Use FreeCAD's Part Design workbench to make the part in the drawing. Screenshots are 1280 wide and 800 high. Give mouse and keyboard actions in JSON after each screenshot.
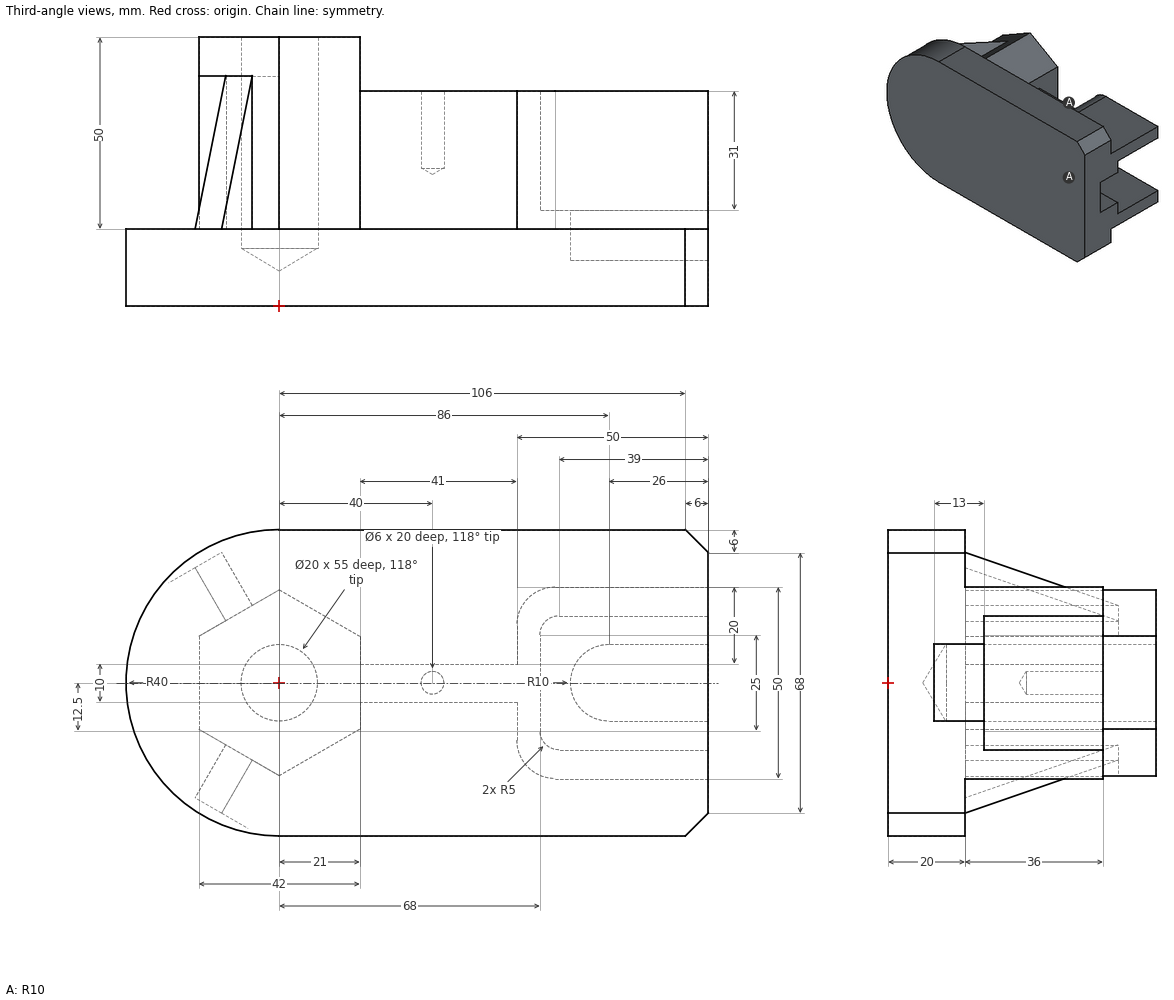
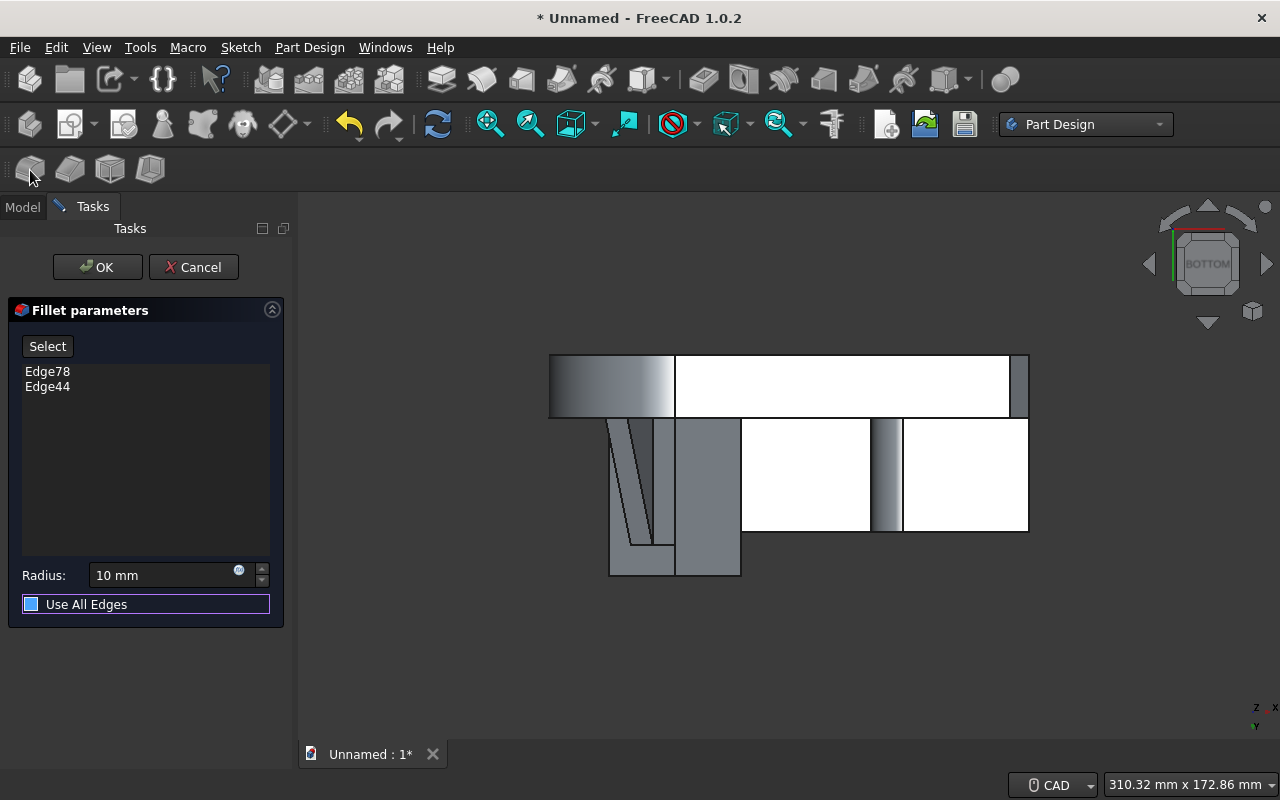
{"action": "left_click", "coordinate": [98, 267]}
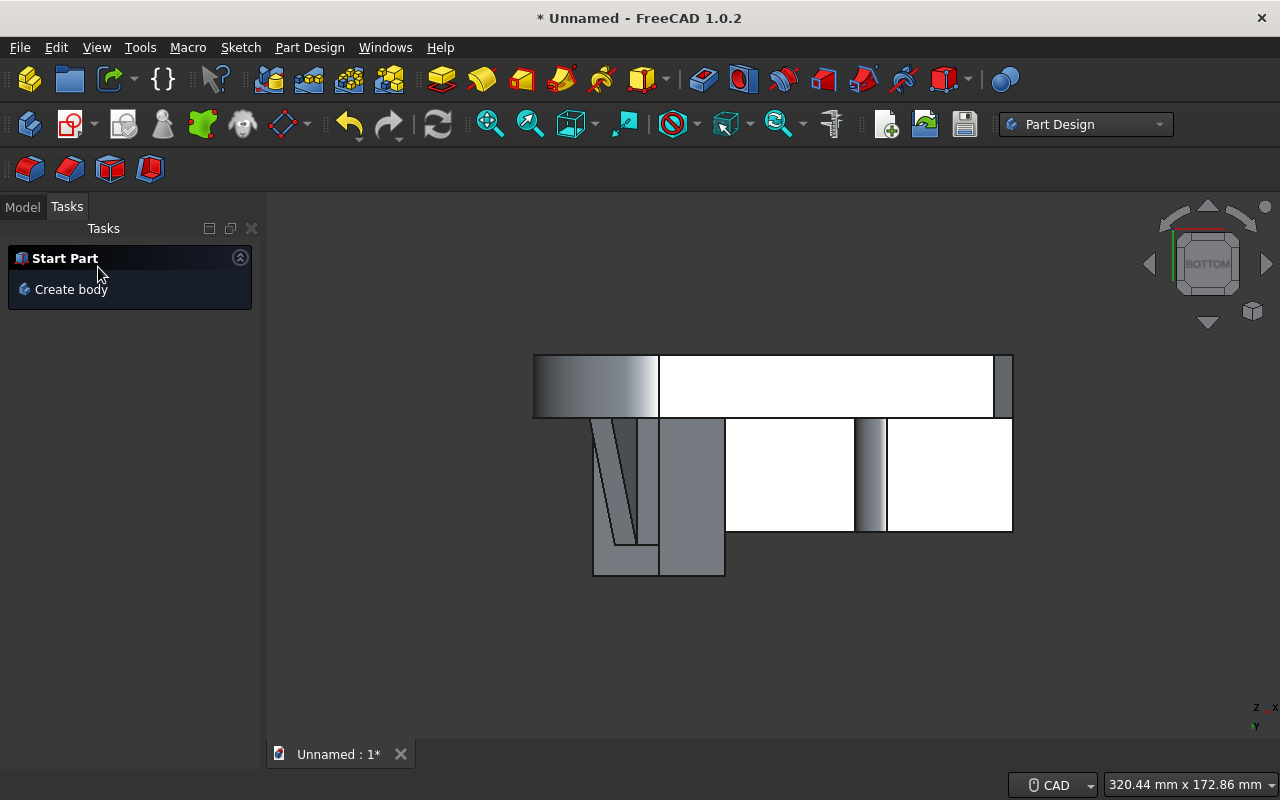
{"action": "key", "text": "4"}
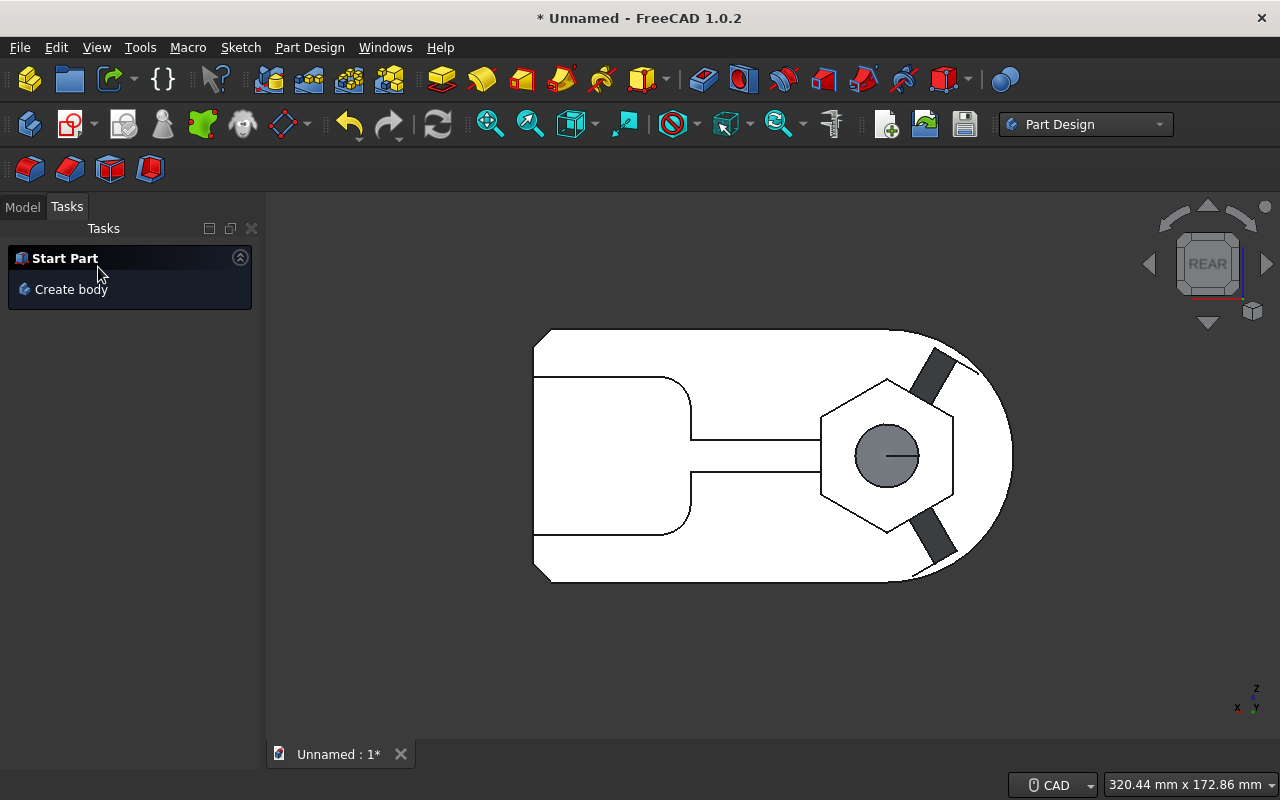
{"action": "left_click", "coordinate": [594, 455]}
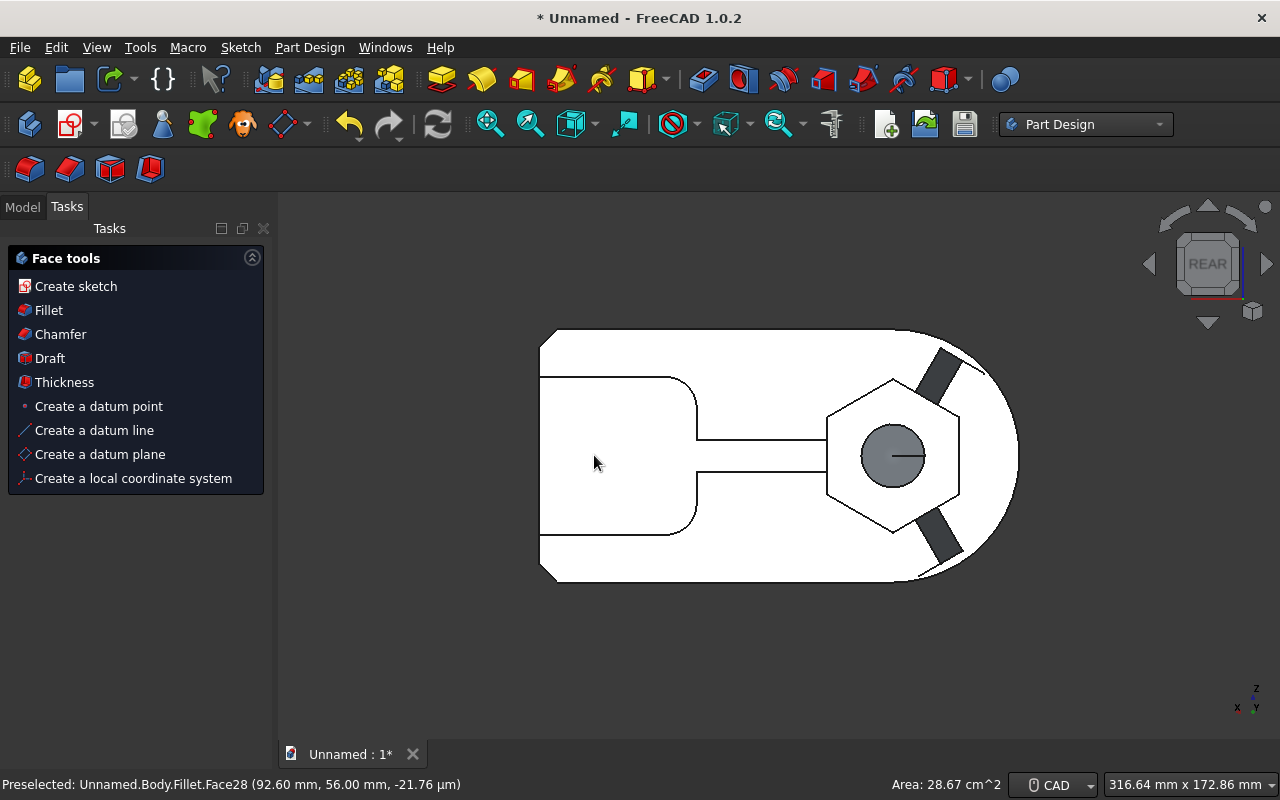
{"action": "left_click", "coordinate": [70, 124]}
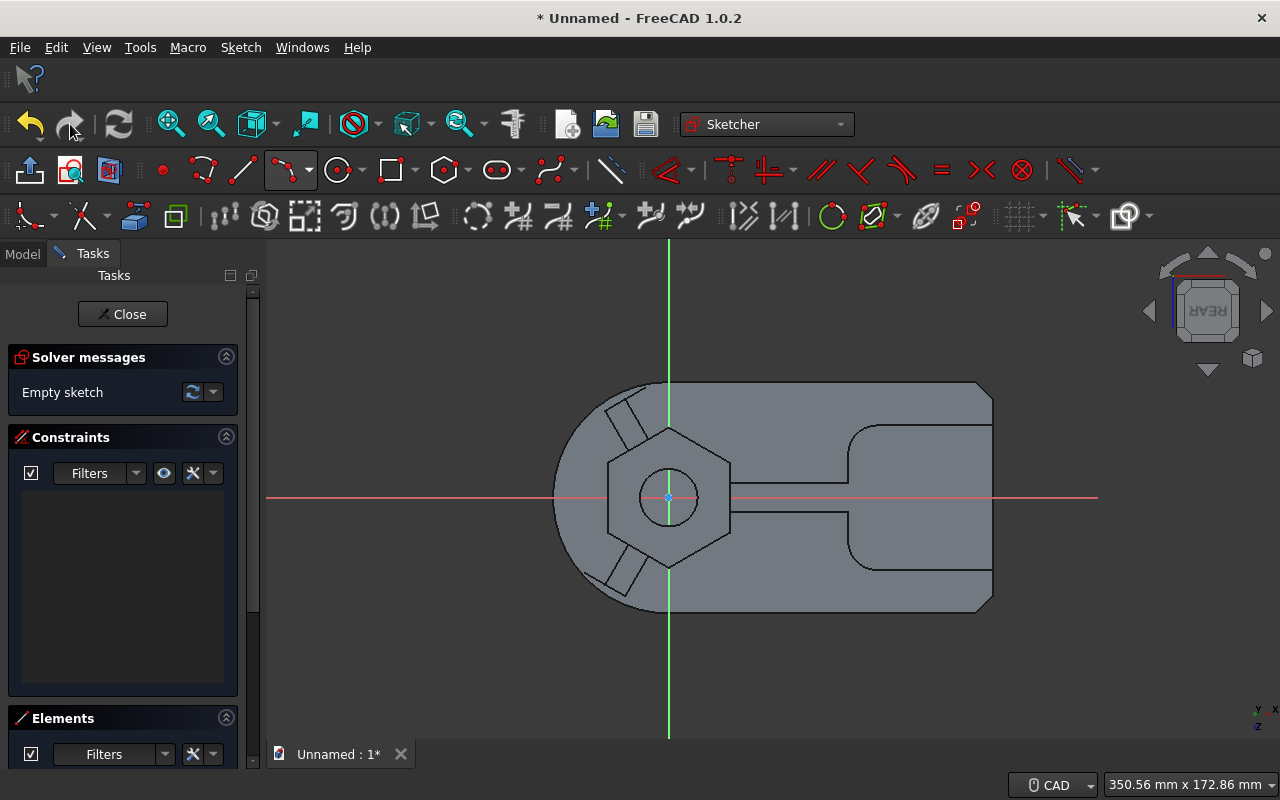
{"action": "scroll", "coordinate": [1026, 502], "scroll_direction": "up", "scroll_amount": 6}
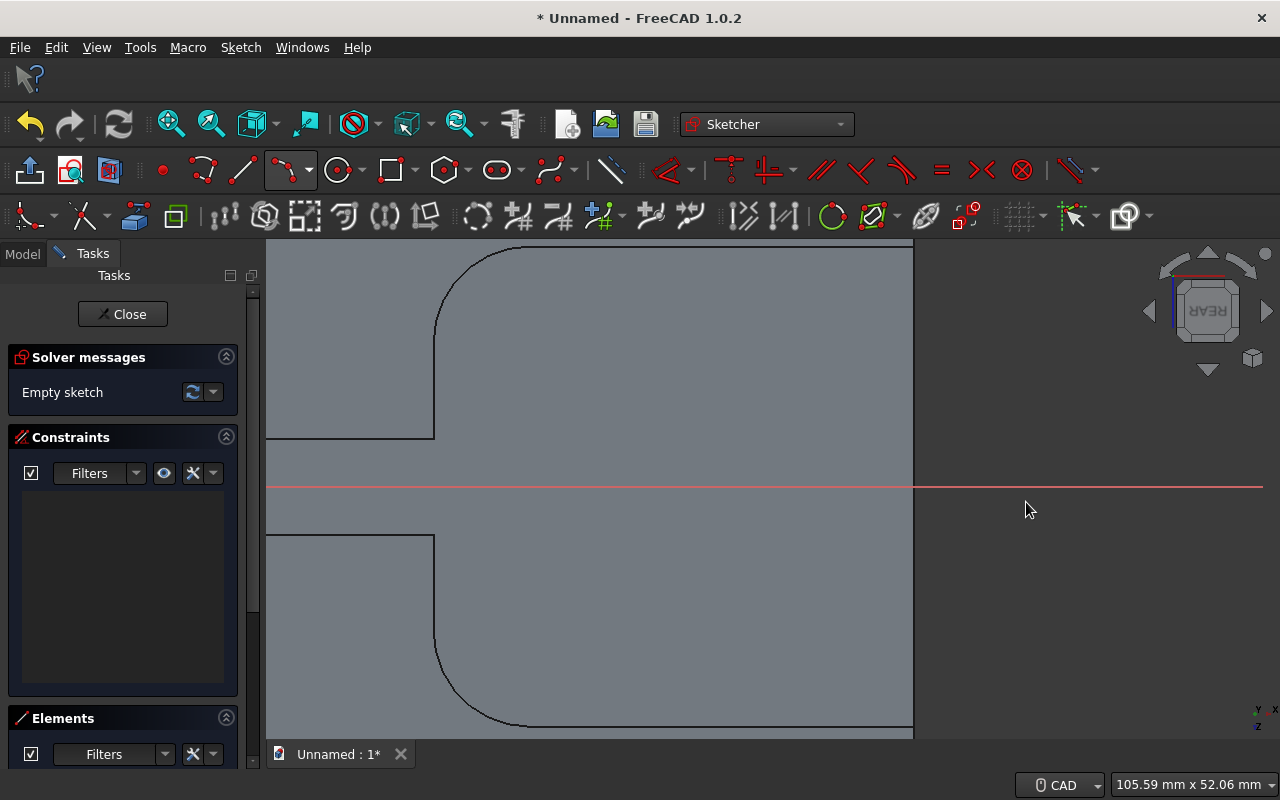
{"action": "left_click", "coordinate": [244, 170]}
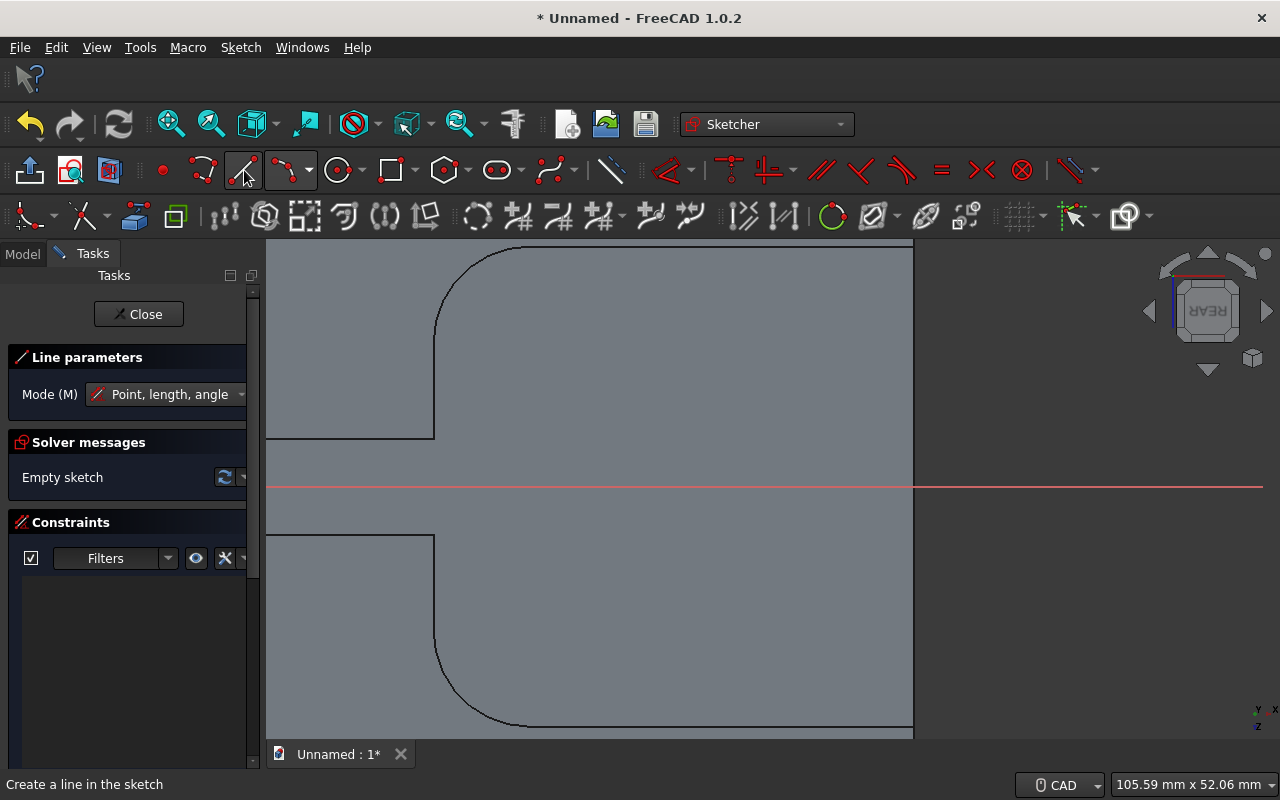
{"action": "left_click", "coordinate": [491, 367]}
{"action": "left_click", "coordinate": [491, 607]}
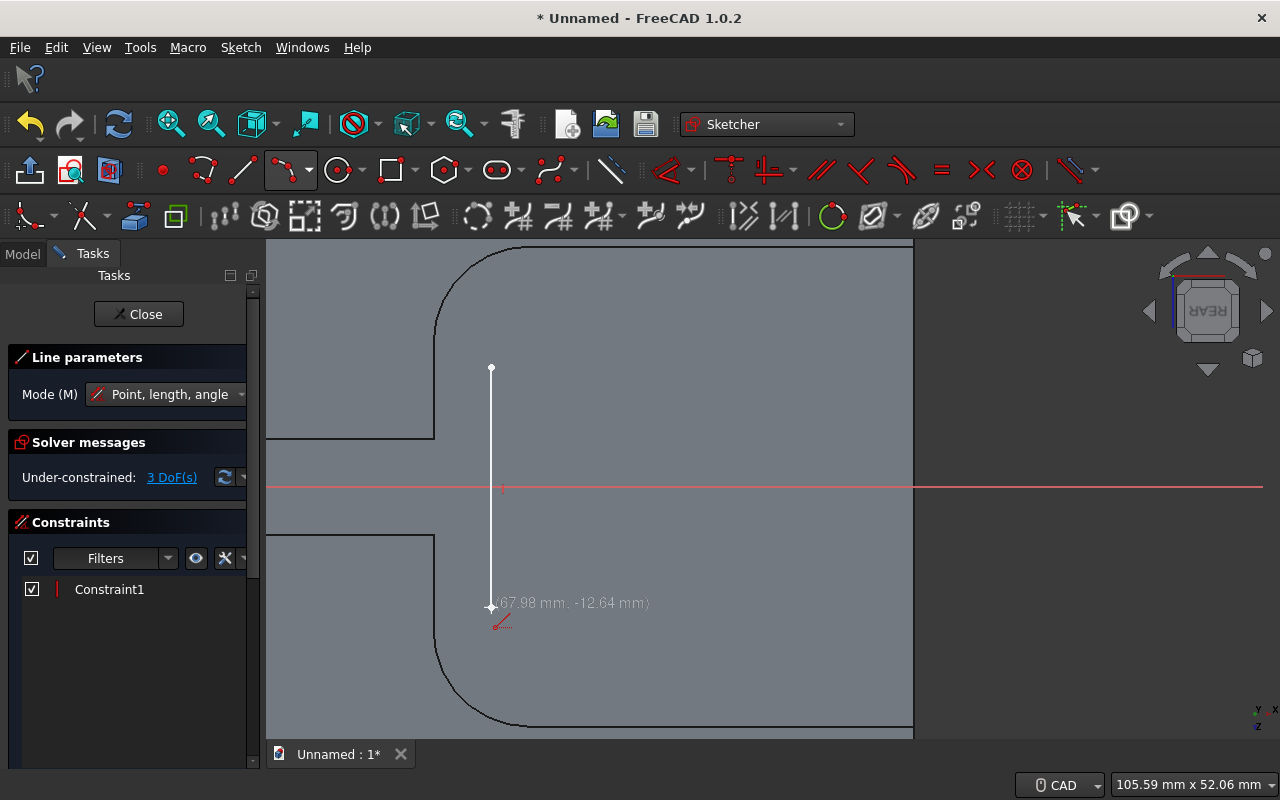
{"action": "left_click", "coordinate": [204, 170]}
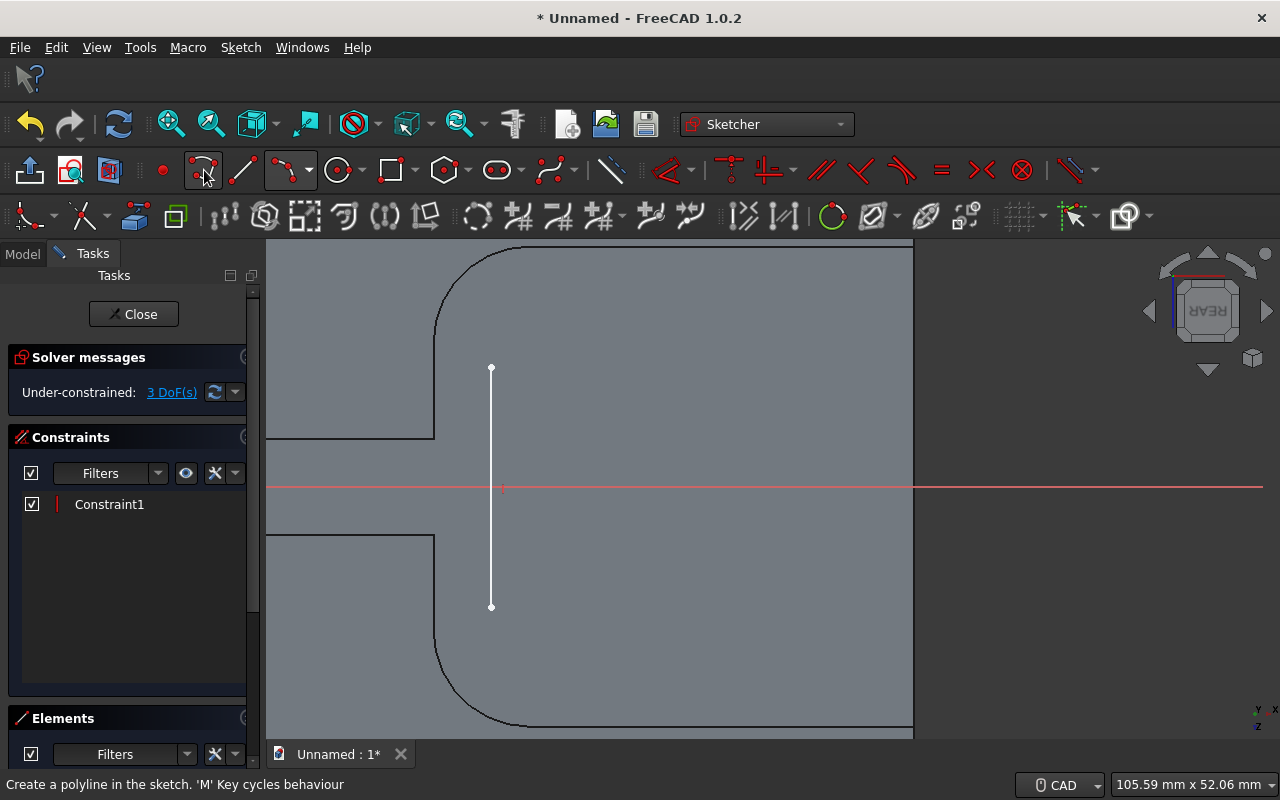
{"action": "left_click", "coordinate": [539, 655]}
{"action": "left_click", "coordinate": [914, 655]}
{"action": "left_click", "coordinate": [914, 319]}
{"action": "left_click", "coordinate": [539, 319]}
{"action": "right_click", "coordinate": [539, 319]}